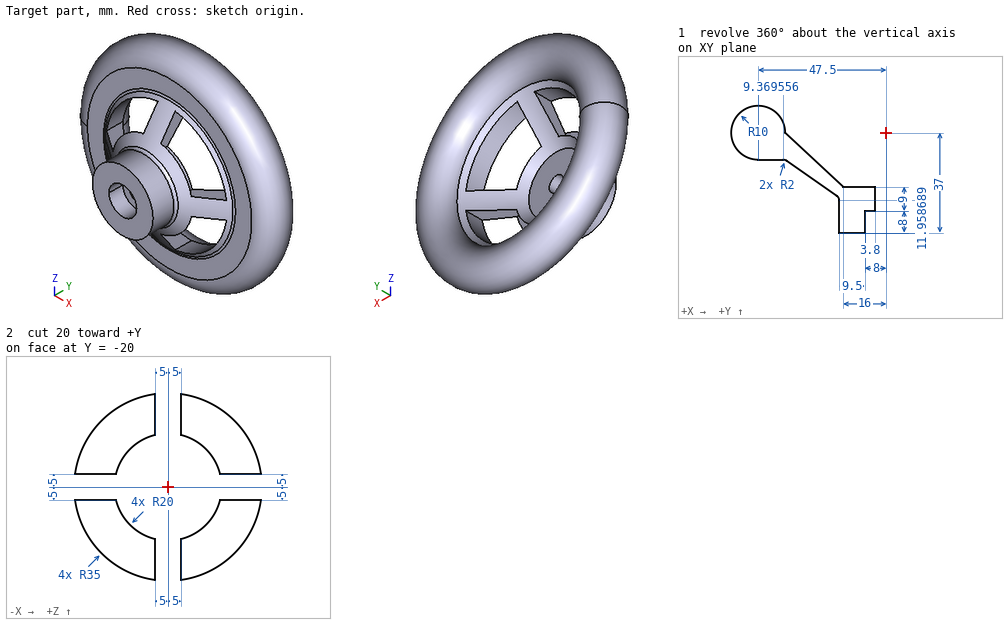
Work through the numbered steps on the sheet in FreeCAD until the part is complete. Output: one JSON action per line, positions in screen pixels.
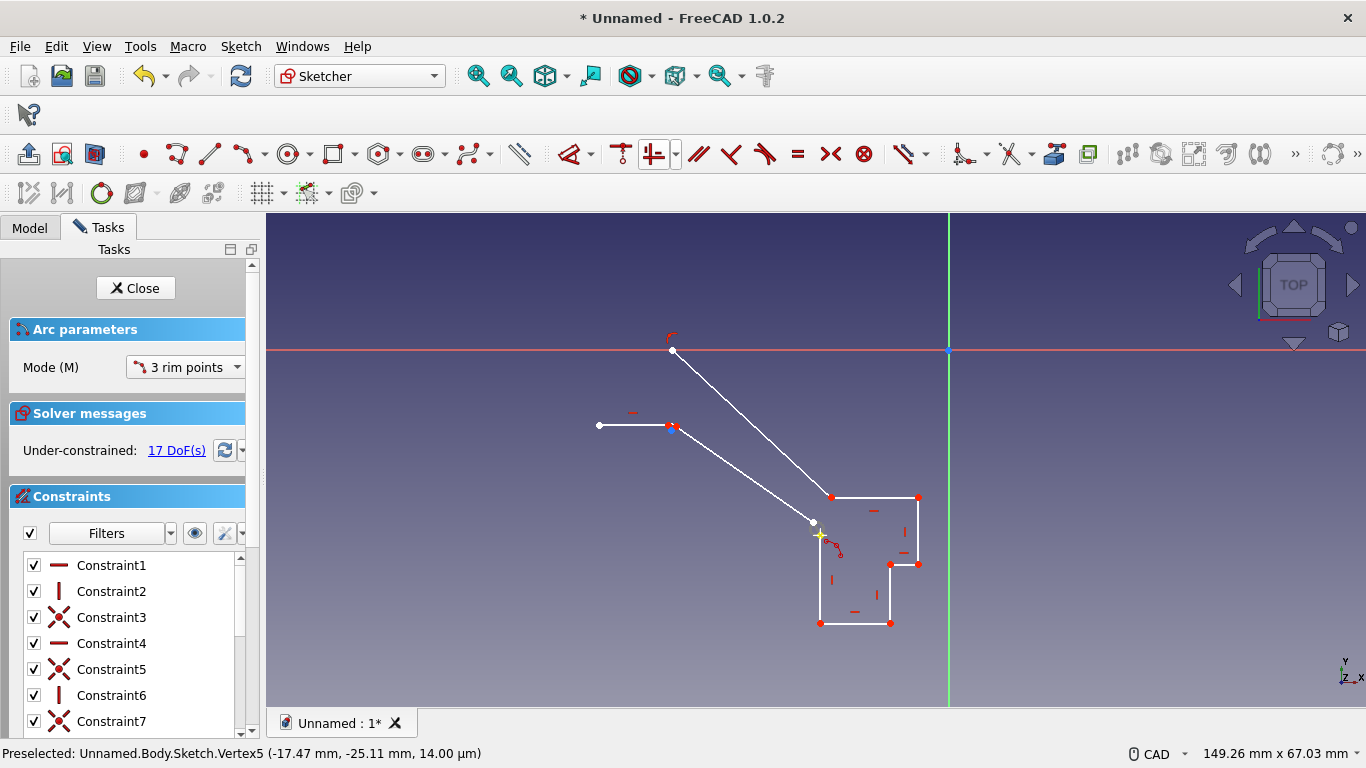
{"action": "scroll", "coordinate": [818, 528], "scroll_direction": "up", "scroll_amount": 12}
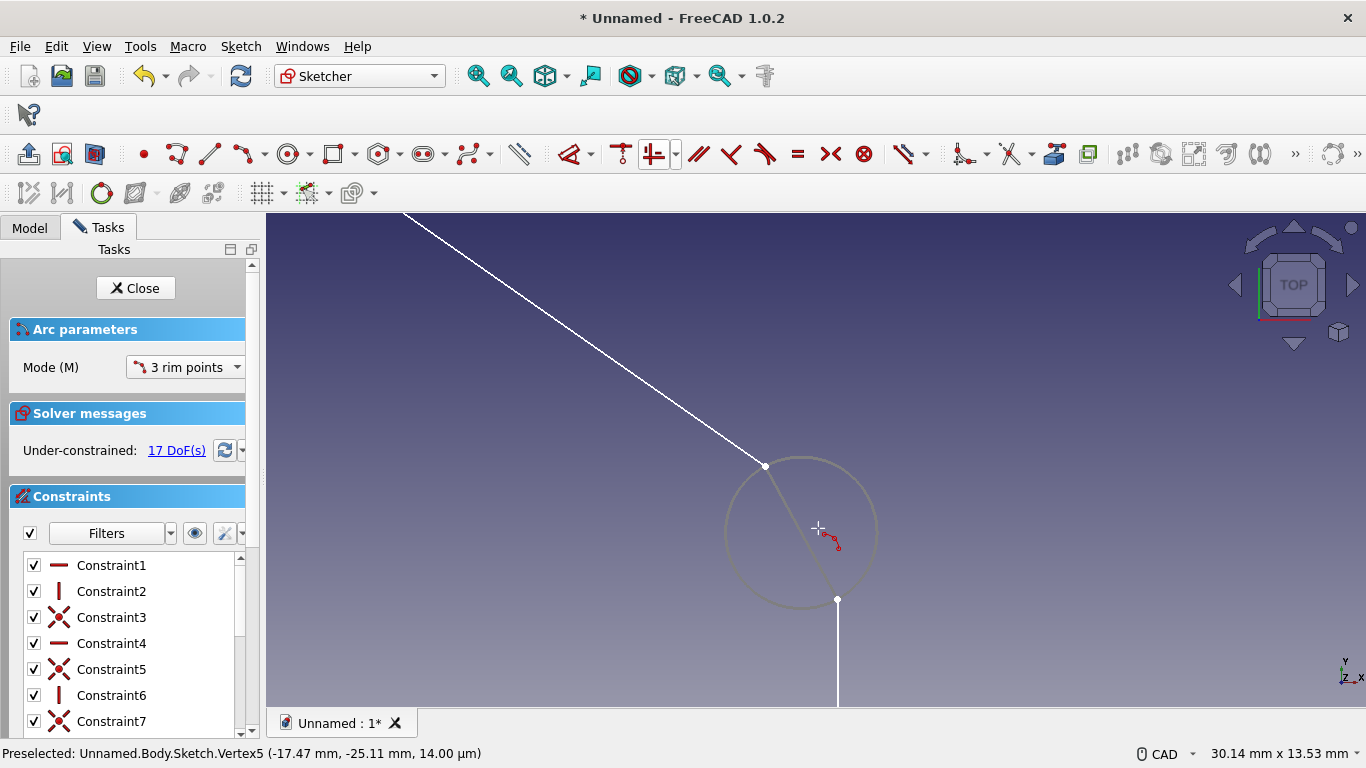
{"action": "left_click", "coordinate": [816, 519]}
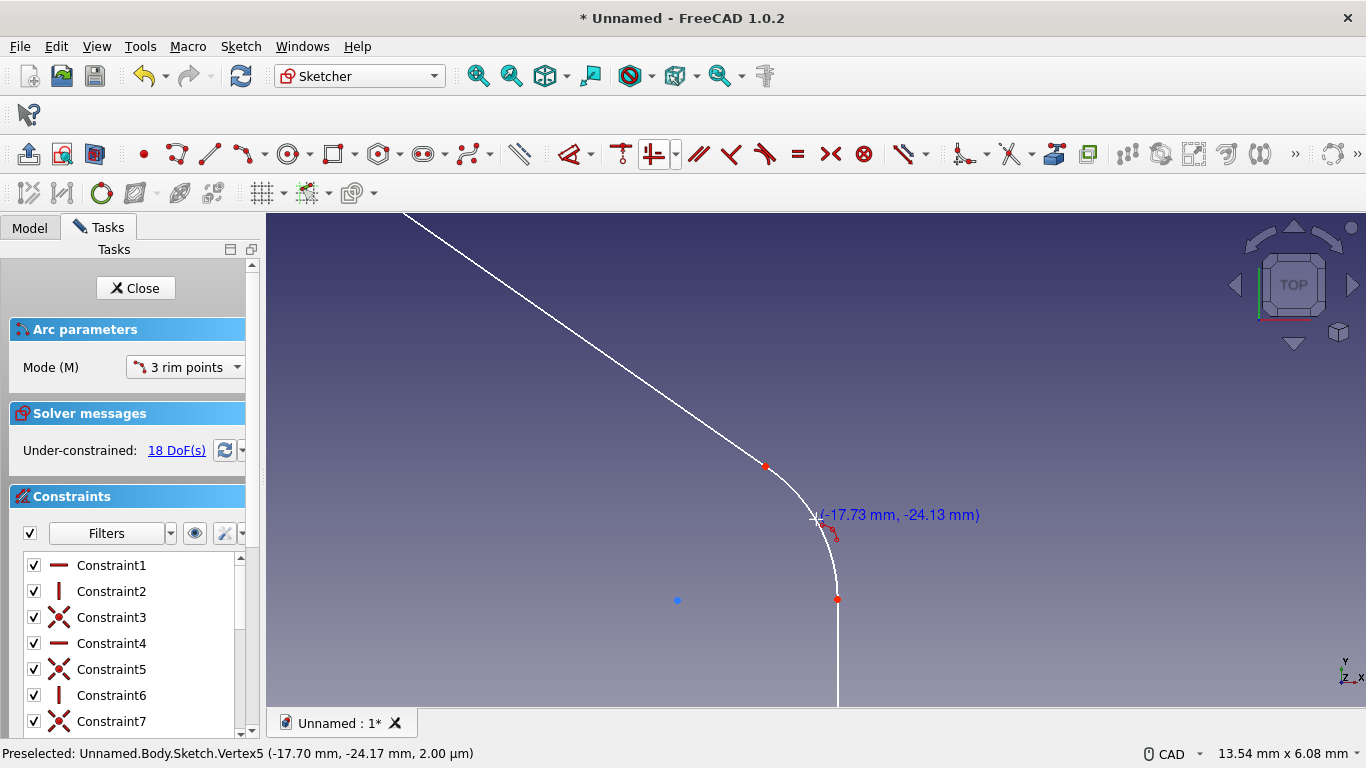
{"action": "scroll", "coordinate": [818, 528], "scroll_direction": "down", "scroll_amount": 12}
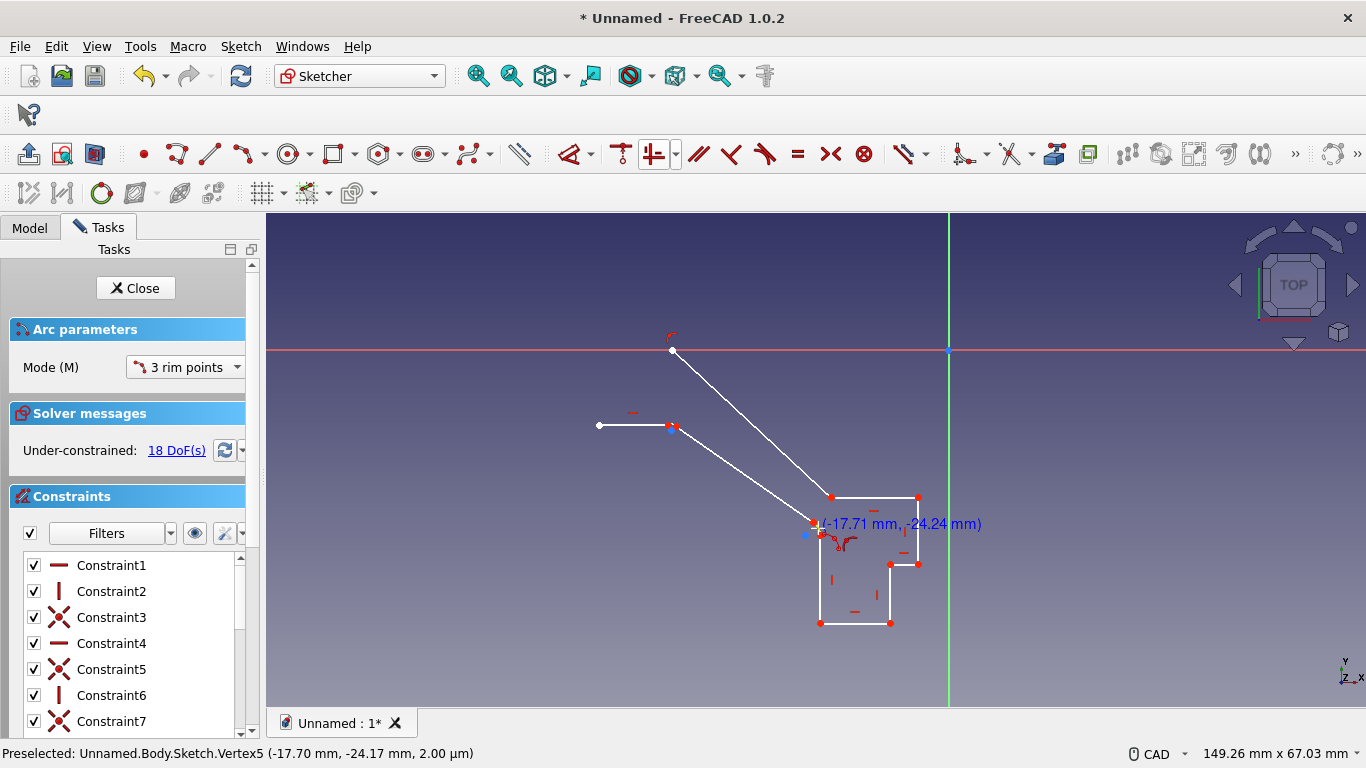
{"action": "left_click", "coordinate": [672, 350]}
{"action": "left_click", "coordinate": [599, 425]}
{"action": "left_click", "coordinate": [547, 298]}
{"action": "key", "text": "Escape"}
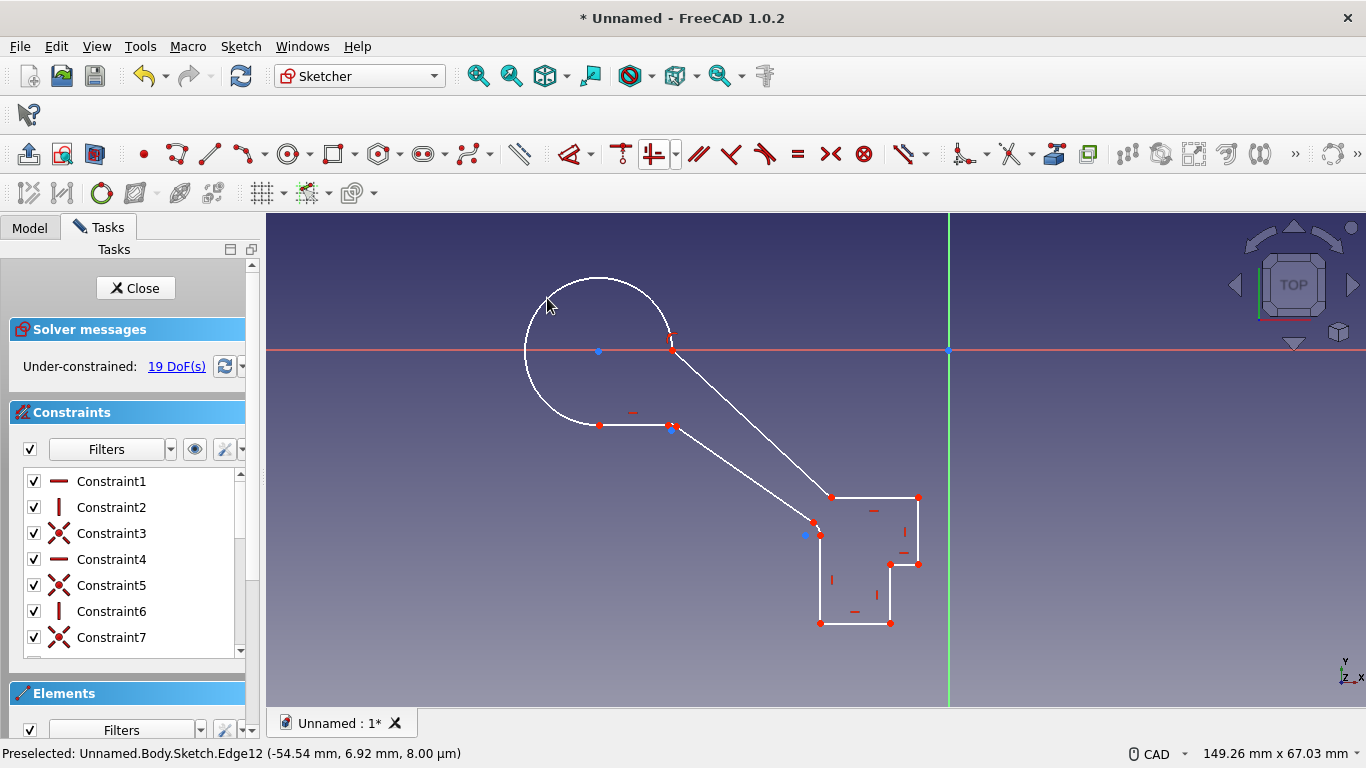
{"action": "left_click", "coordinate": [620, 425]}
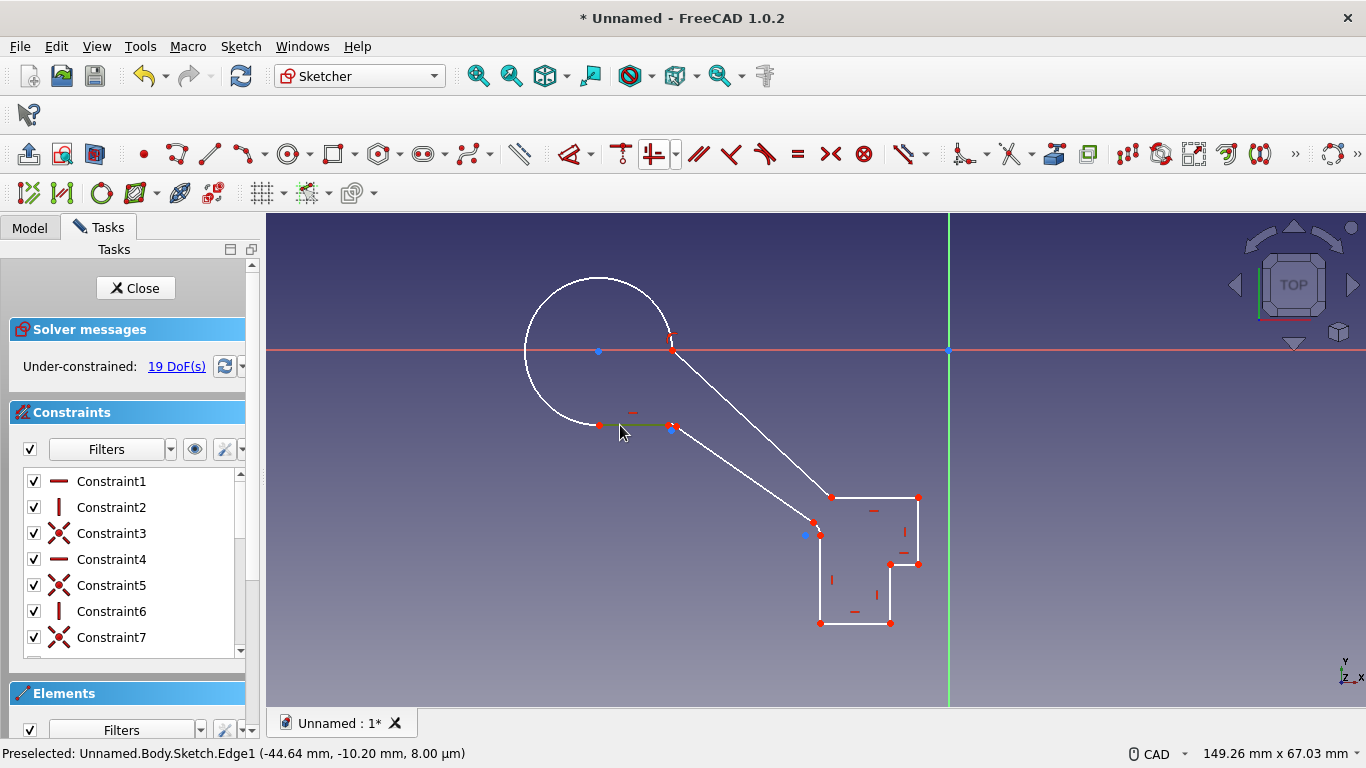
{"action": "scroll", "coordinate": [673, 425], "scroll_direction": "up", "scroll_amount": 6}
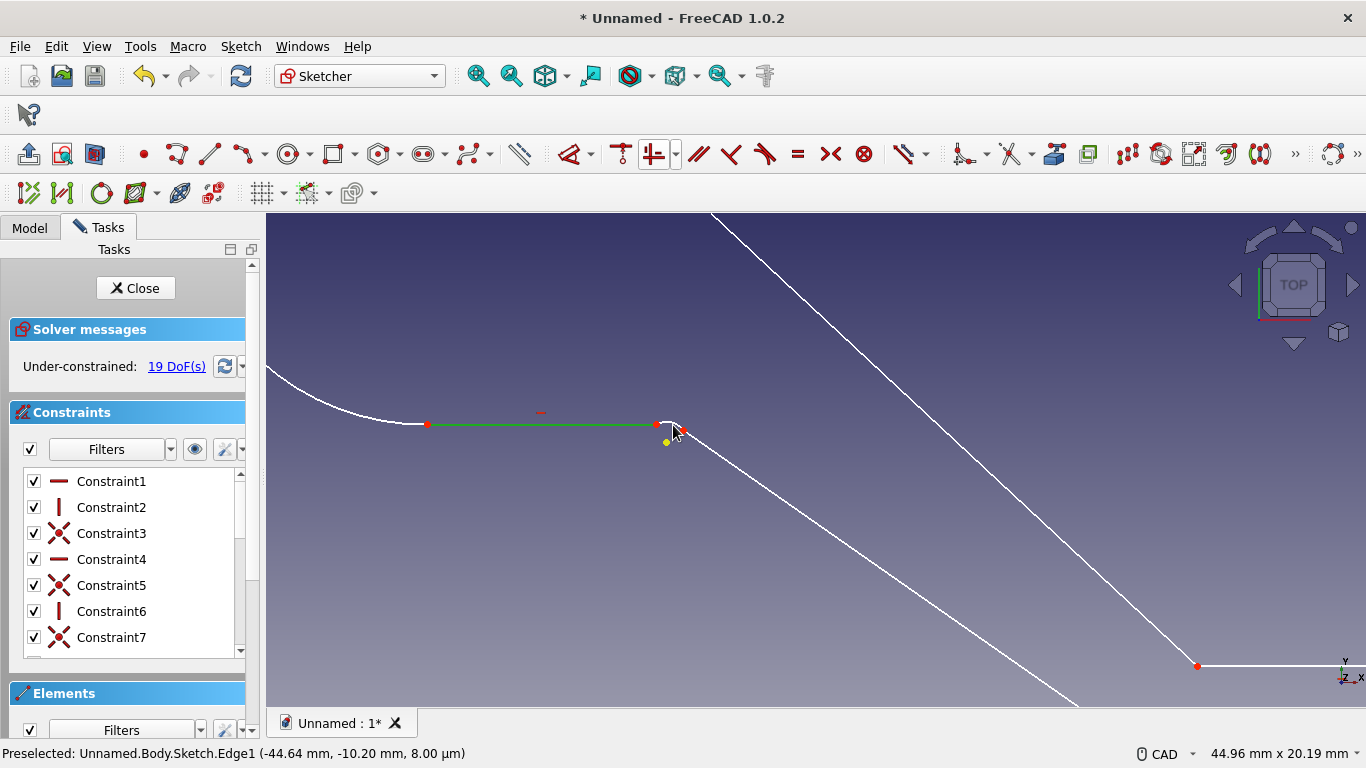
{"action": "left_click", "coordinate": [671, 422]}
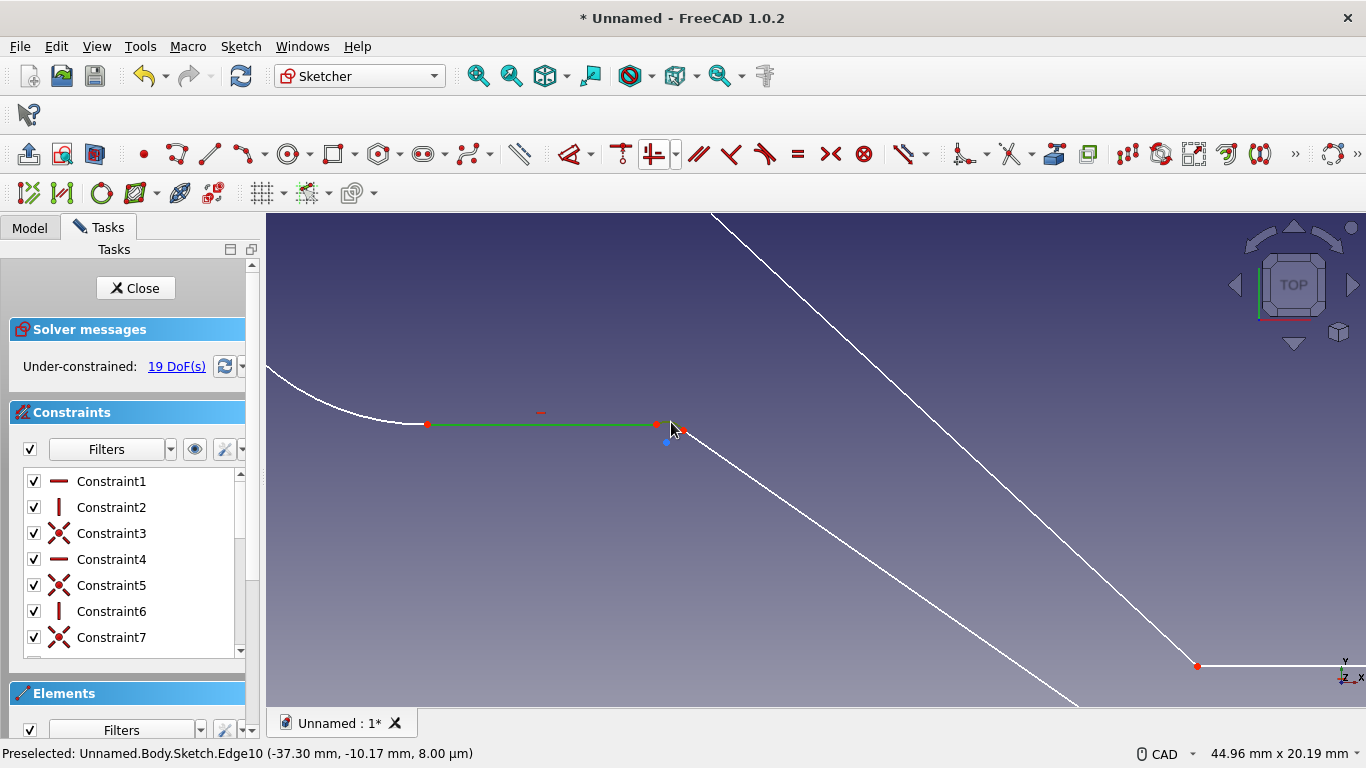
{"action": "left_click", "coordinate": [765, 154]}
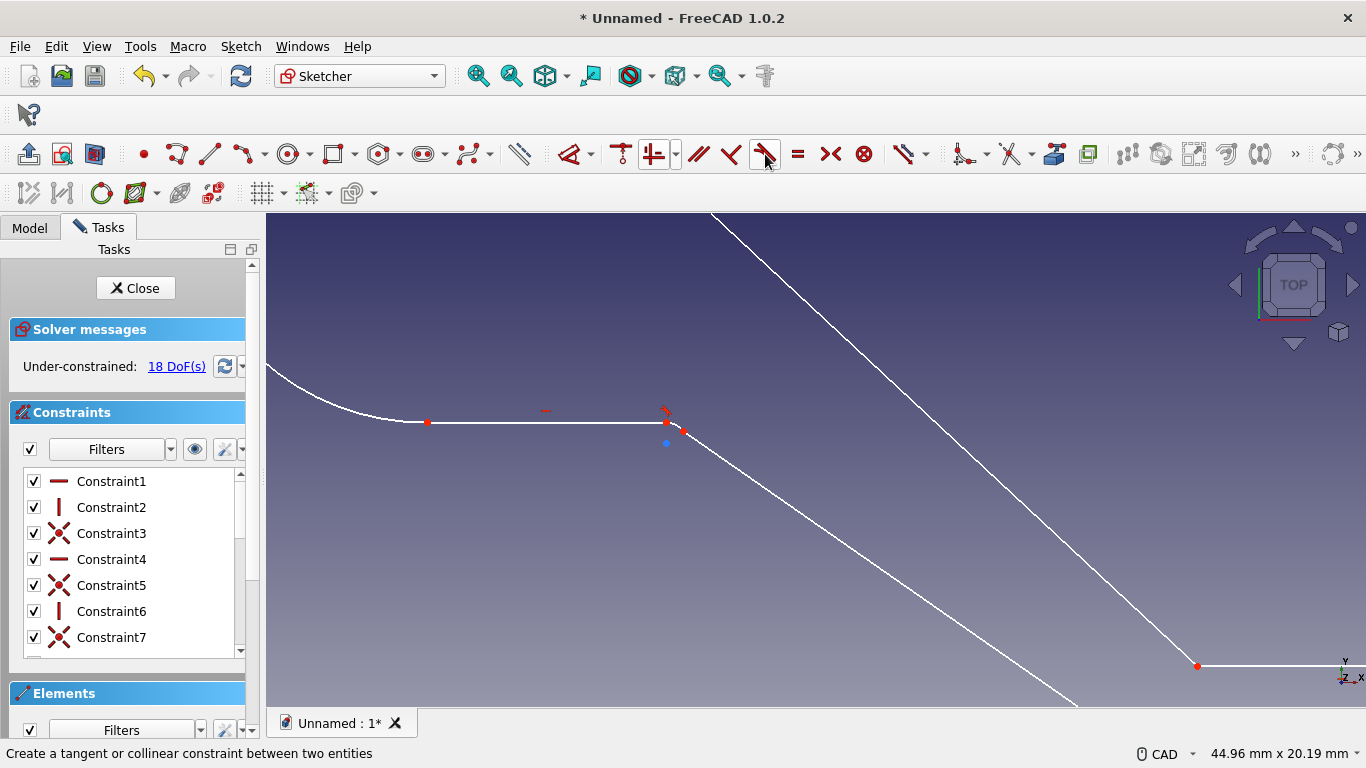
{"action": "left_click", "coordinate": [499, 423]}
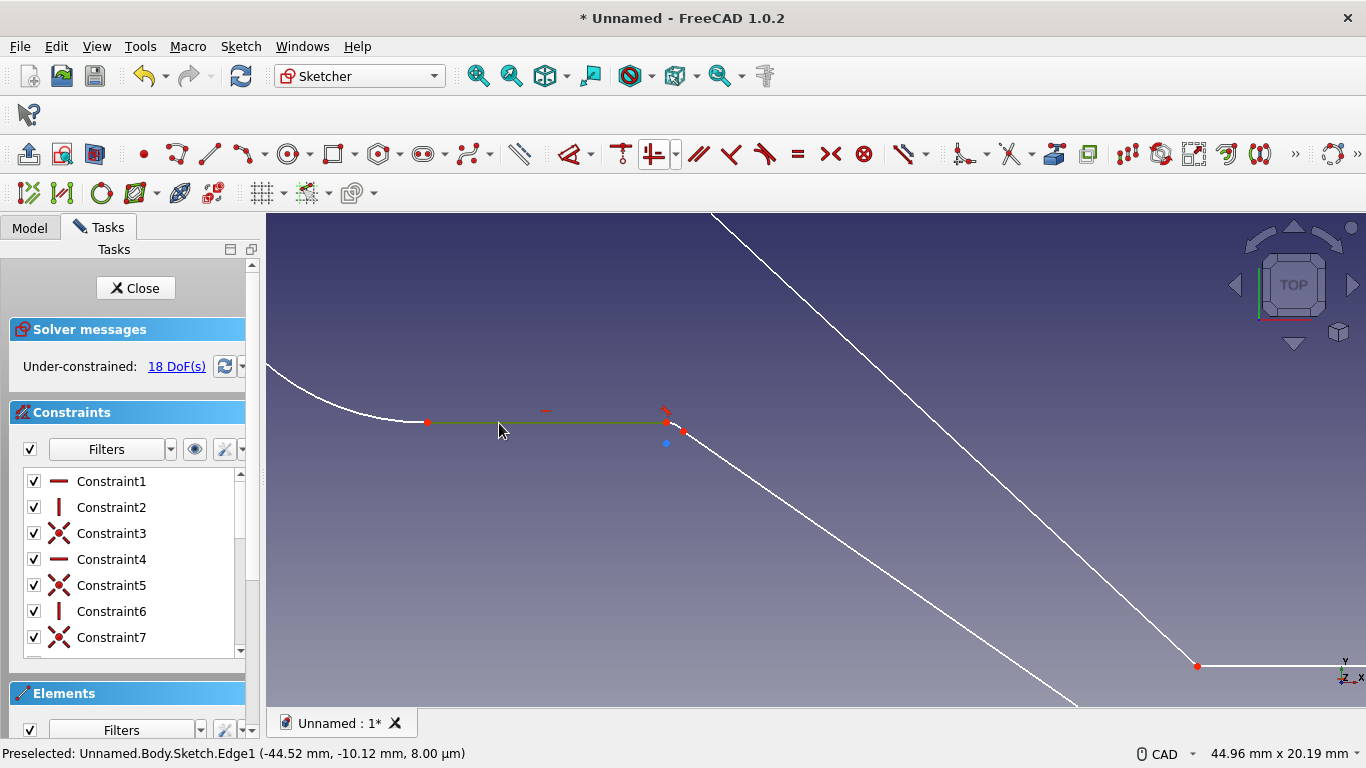
{"action": "scroll", "coordinate": [673, 425], "scroll_direction": "down", "scroll_amount": 6}